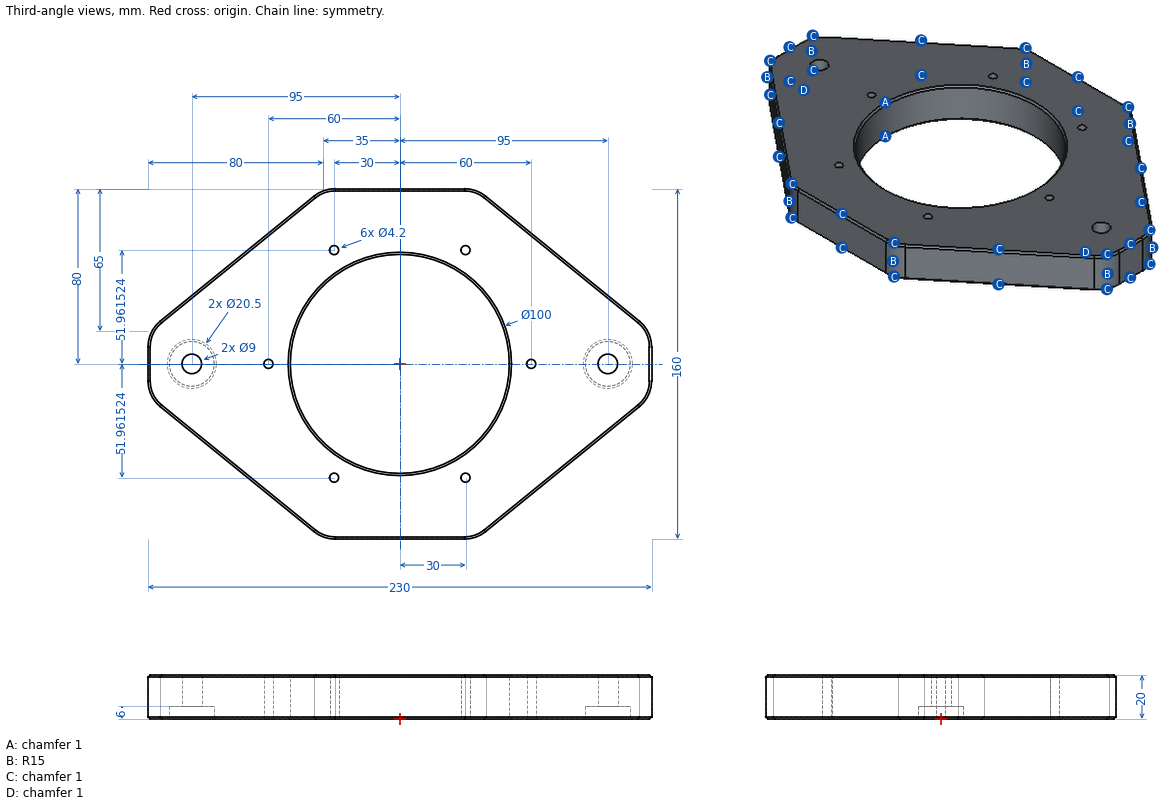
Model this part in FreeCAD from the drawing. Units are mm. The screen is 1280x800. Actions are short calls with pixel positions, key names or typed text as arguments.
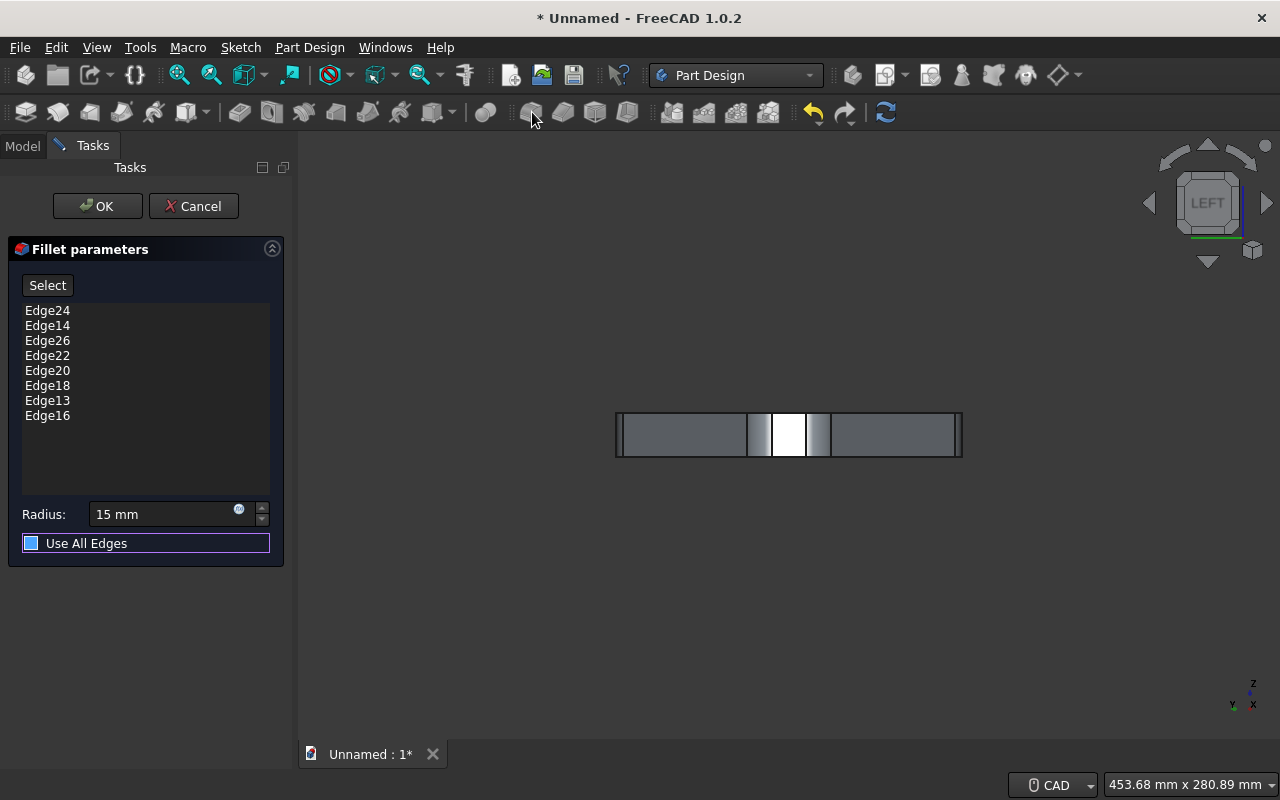
click(98, 206)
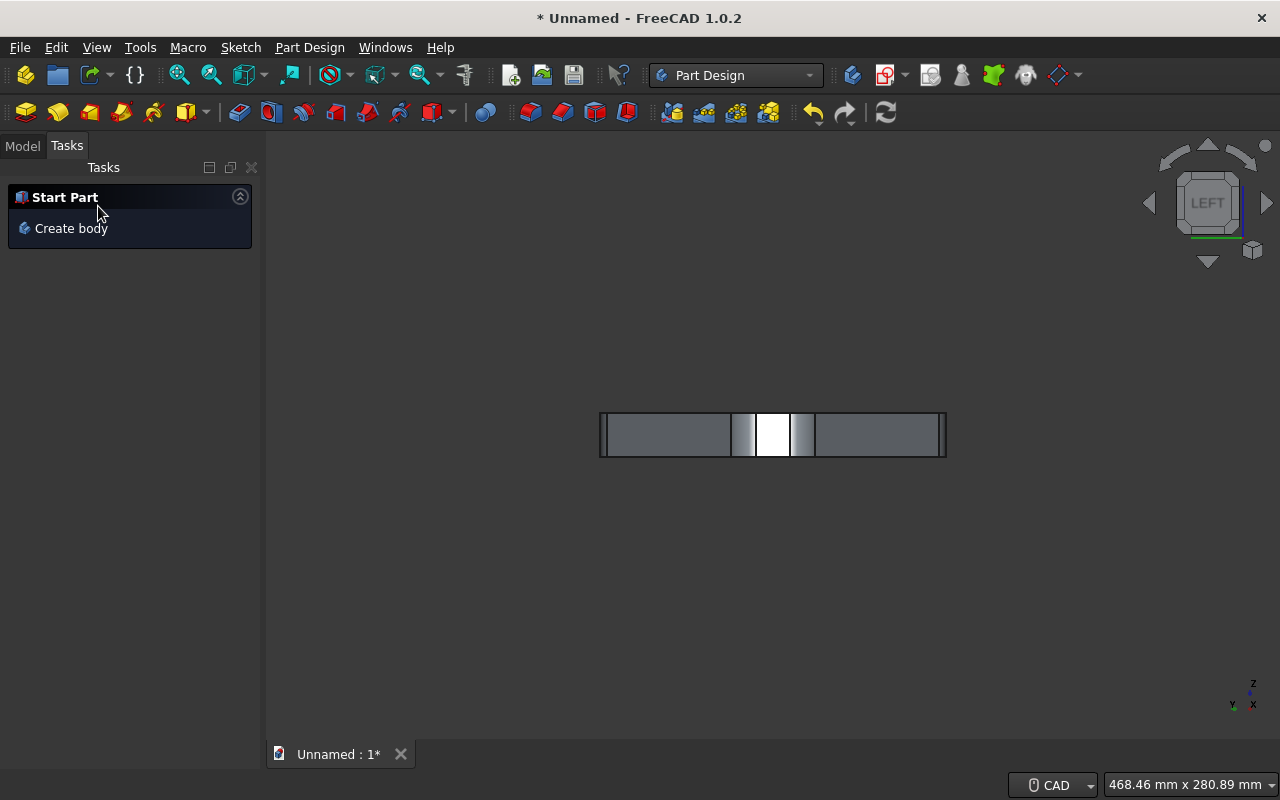
click(180, 76)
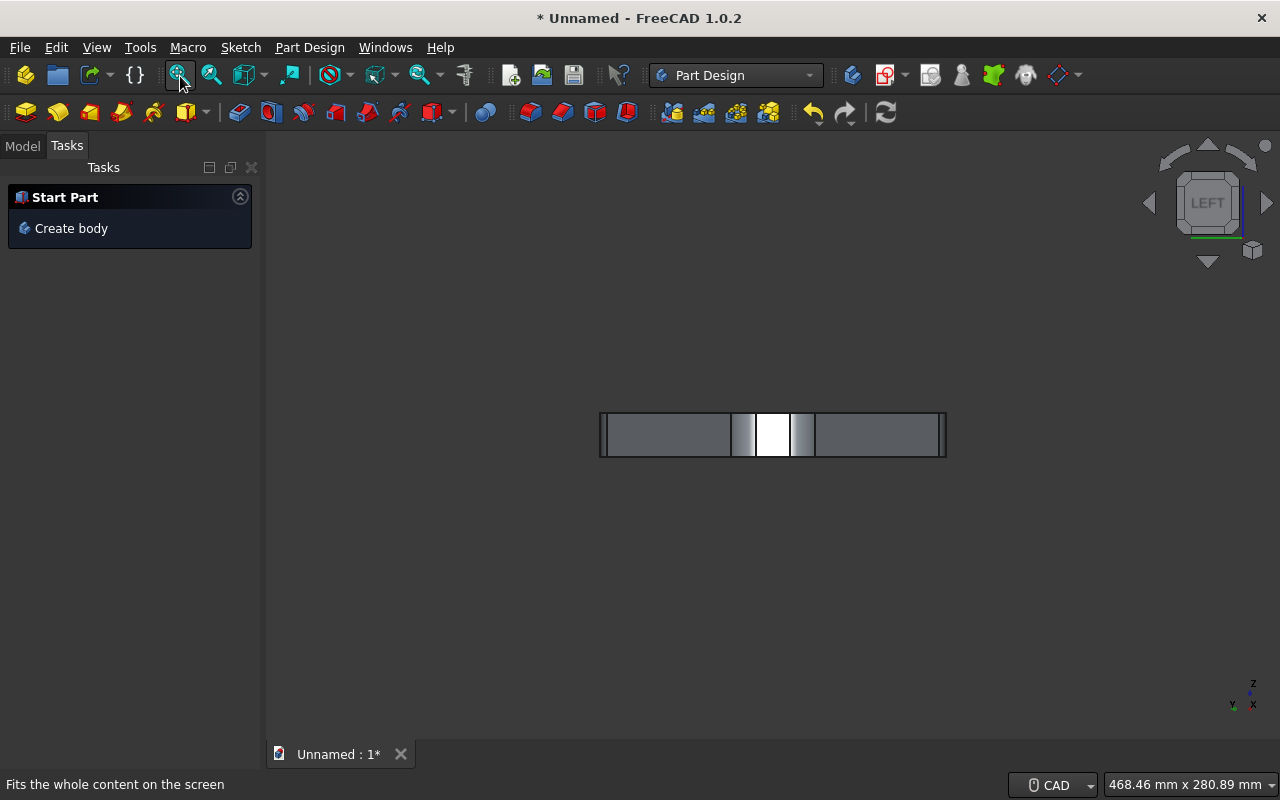
click(669, 456)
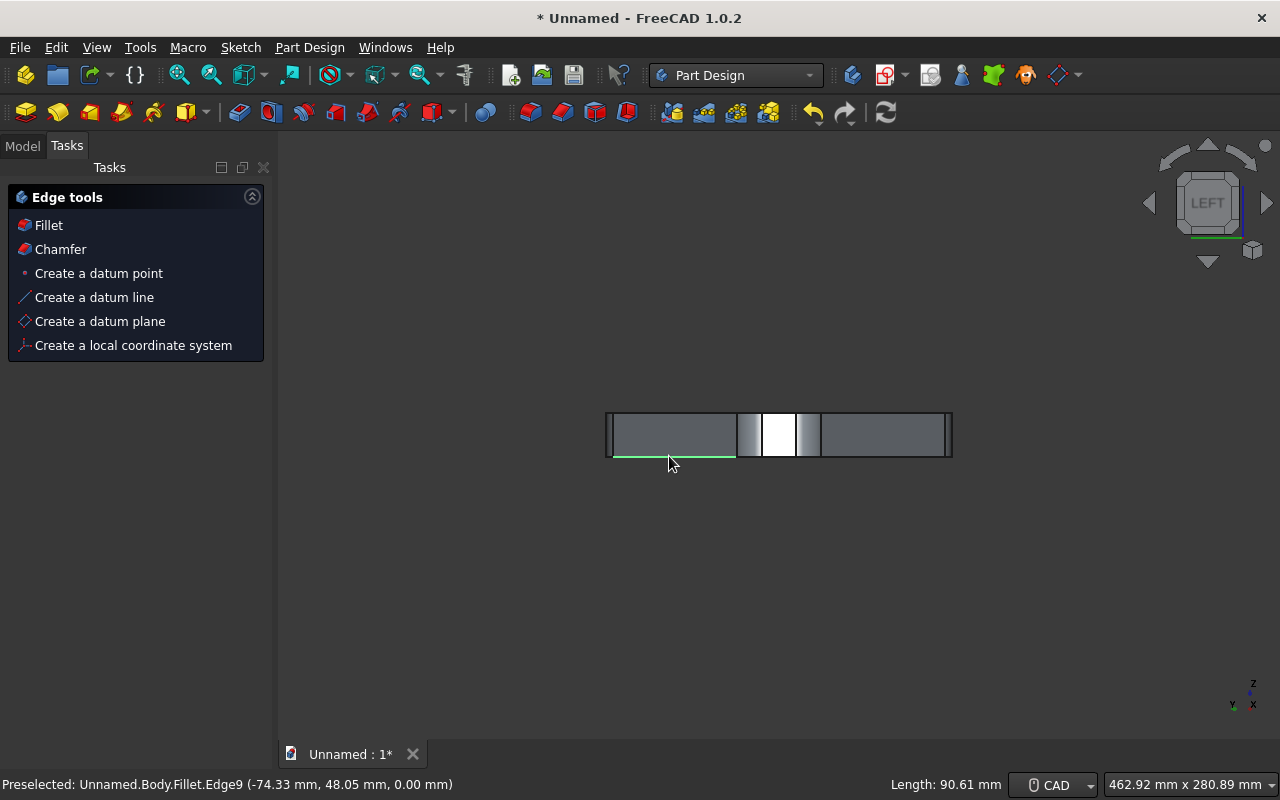
click(675, 412, ctrl)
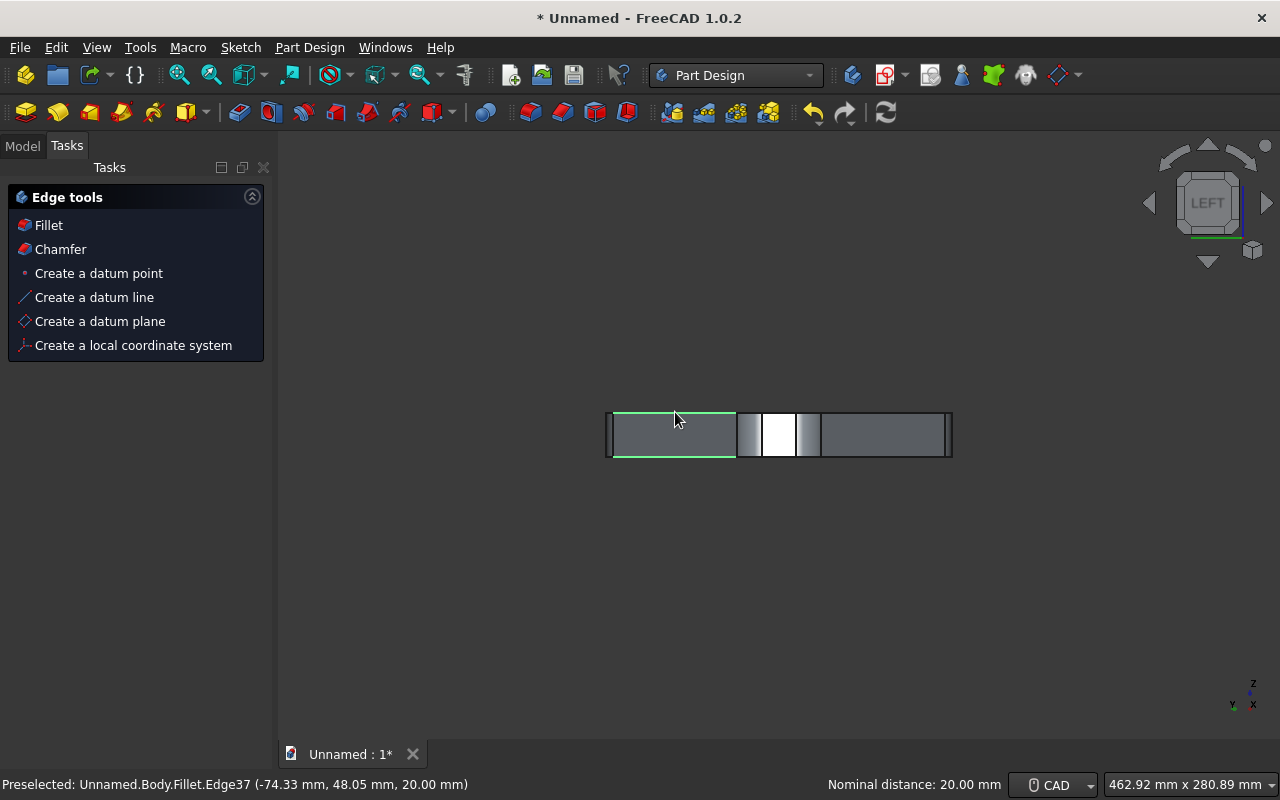
click(779, 412, ctrl)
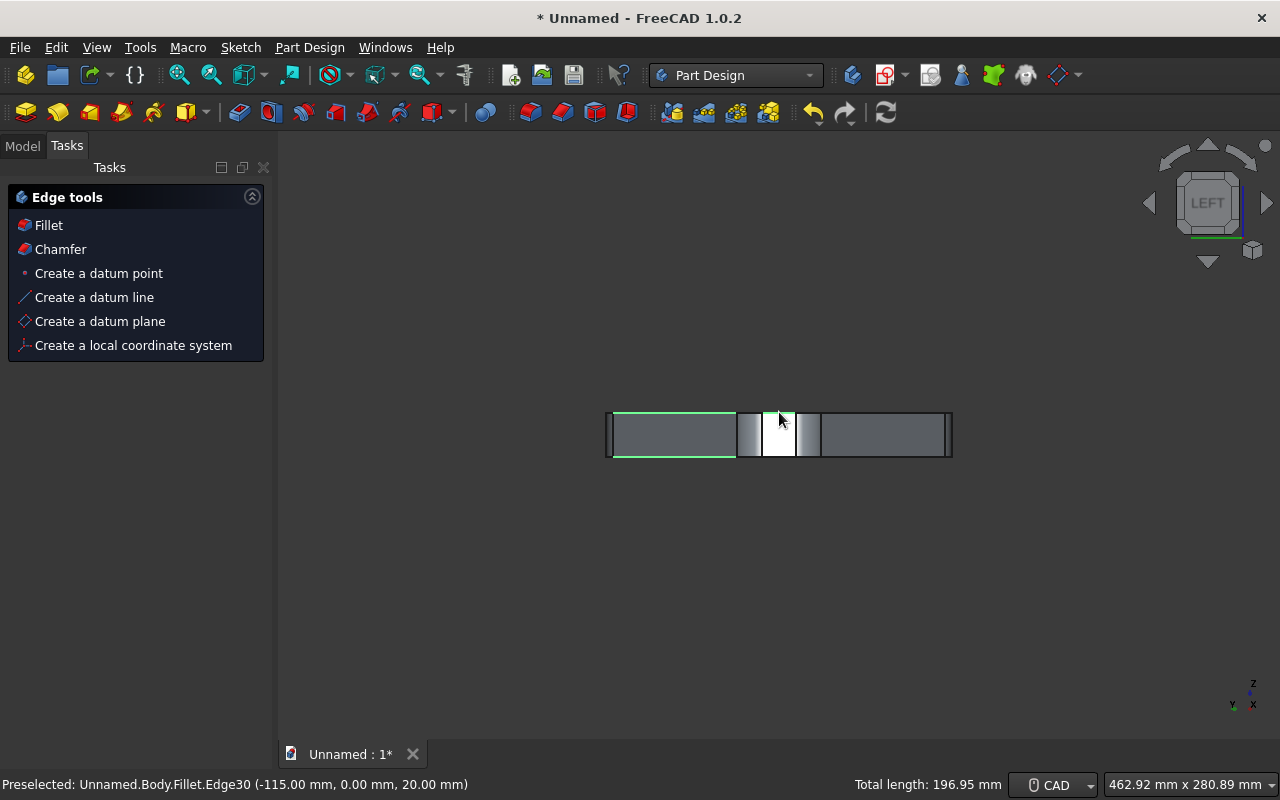
click(883, 412, ctrl)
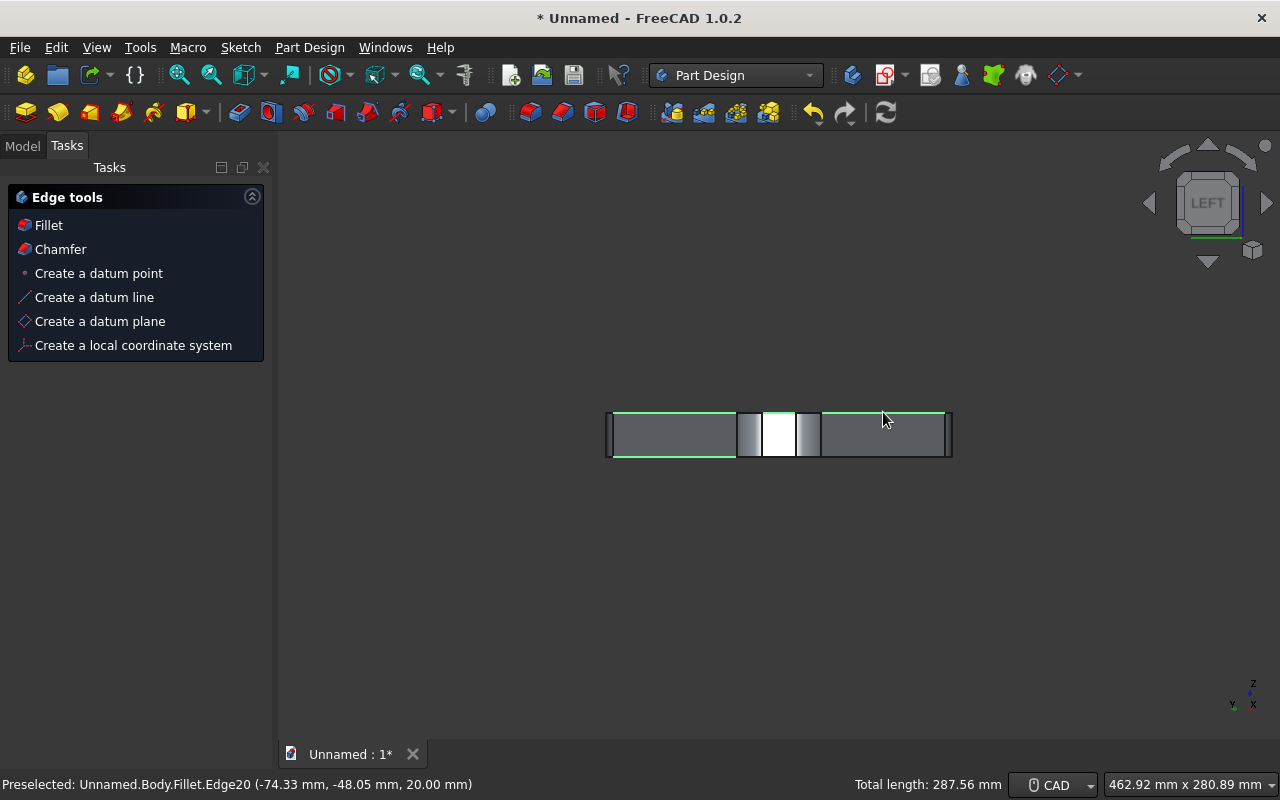
click(810, 412, ctrl)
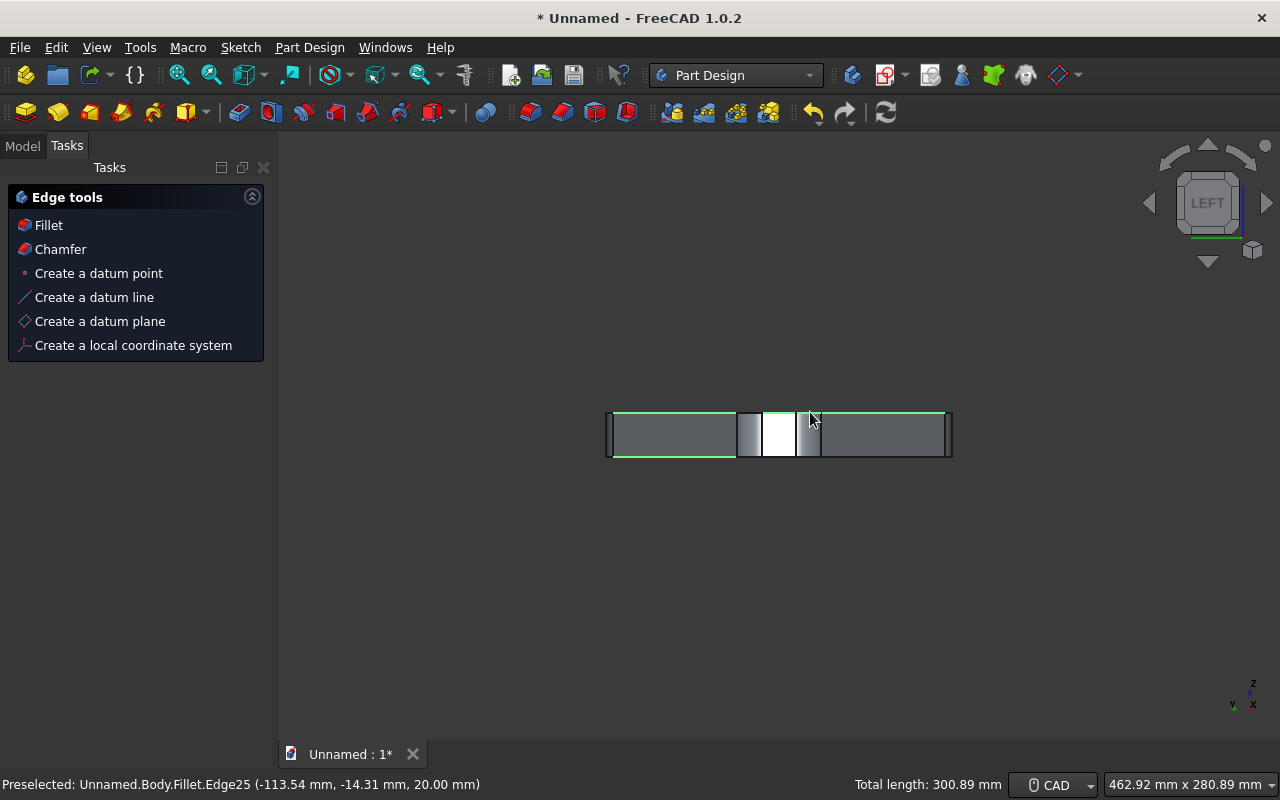
click(951, 412, ctrl)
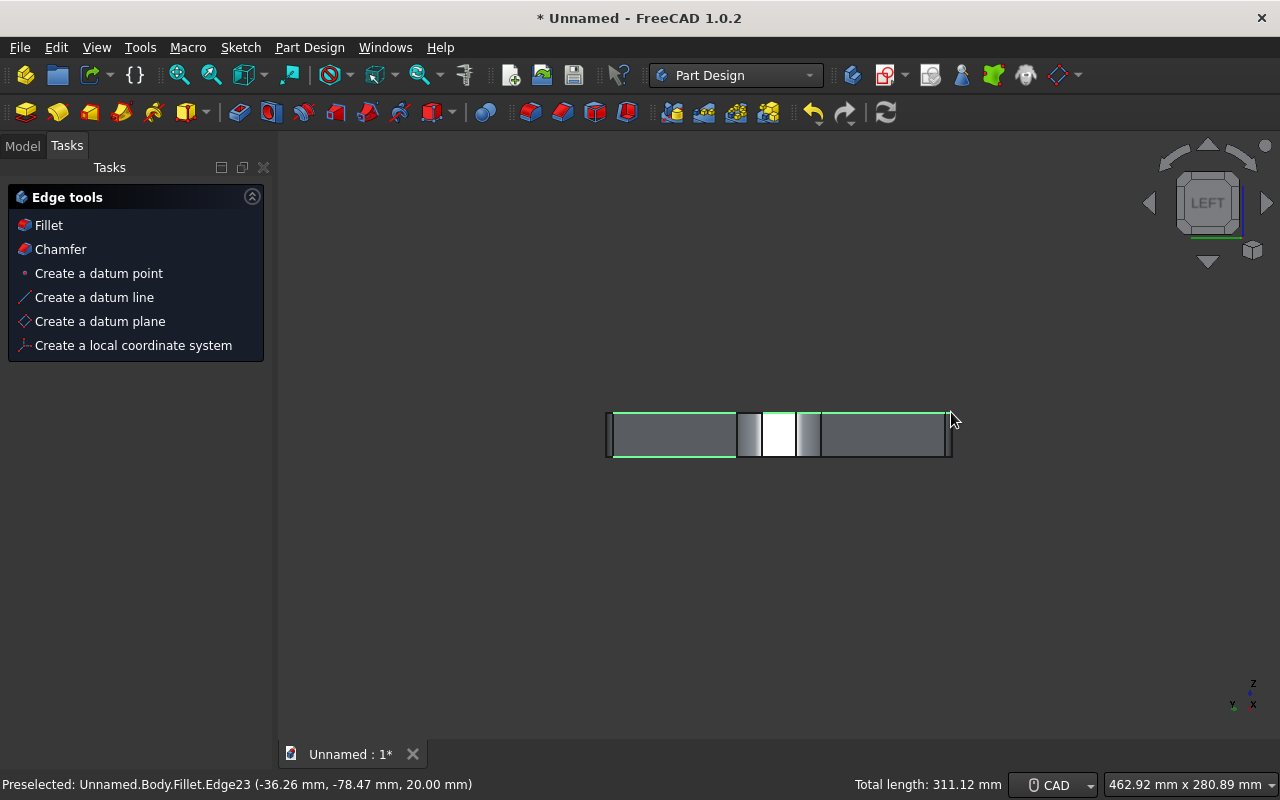
click(607, 412, ctrl)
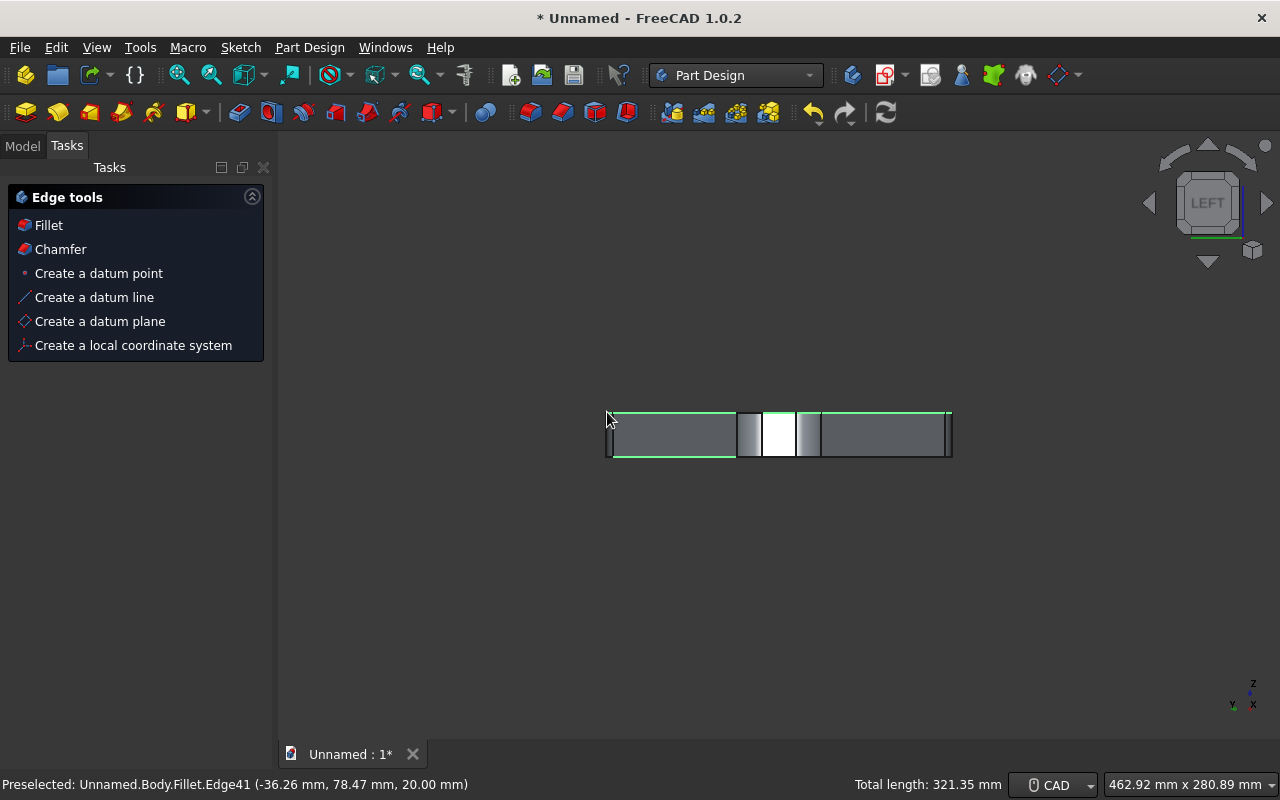
click(748, 412, ctrl)